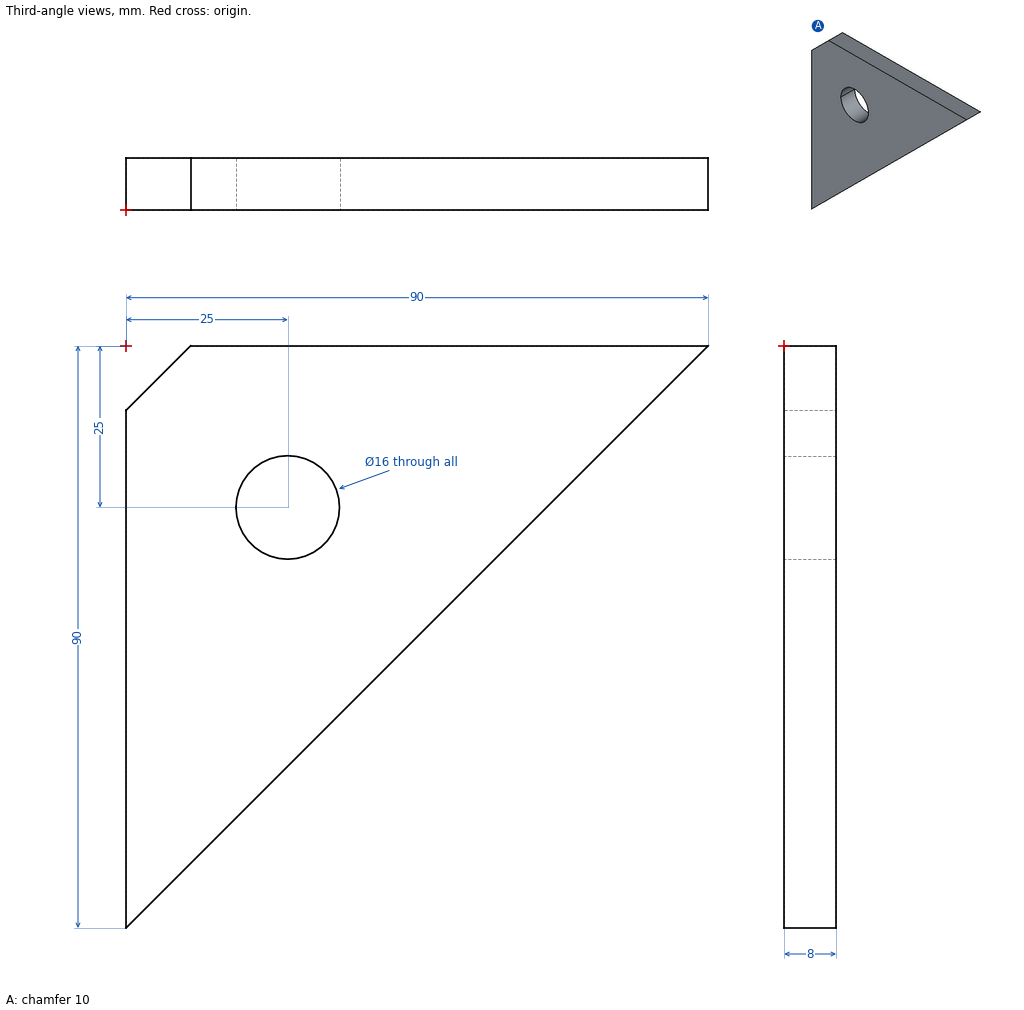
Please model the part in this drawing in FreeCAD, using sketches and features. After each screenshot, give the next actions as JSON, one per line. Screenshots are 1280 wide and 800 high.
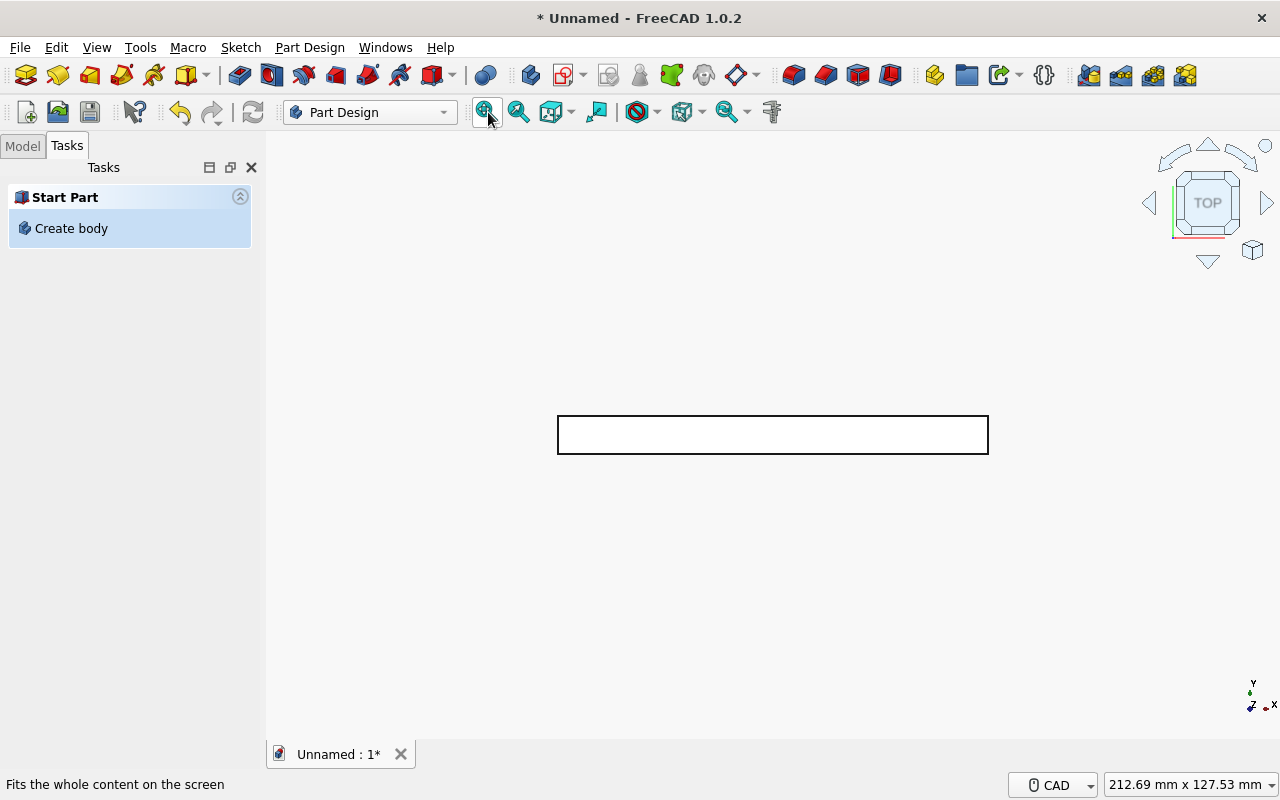
{"action": "left_click", "coordinate": [488, 112]}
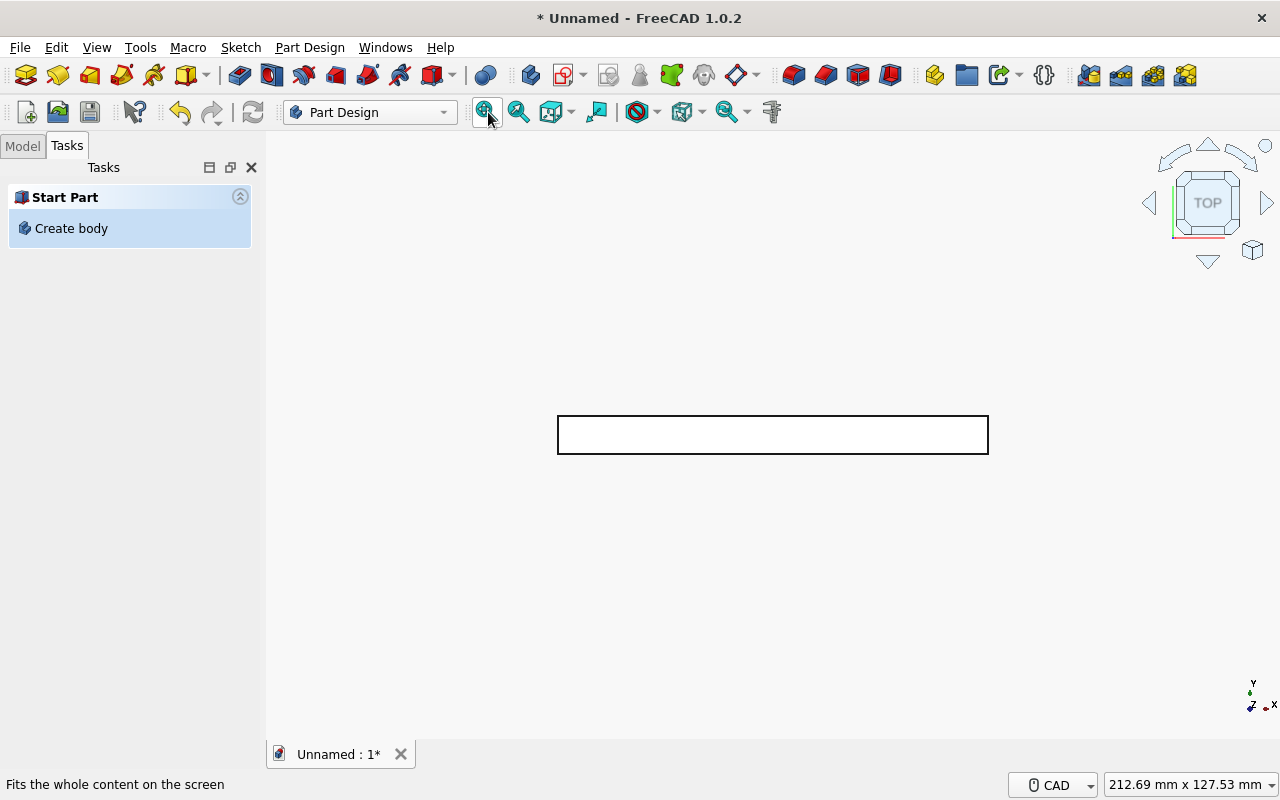
{"action": "left_click", "coordinate": [558, 423]}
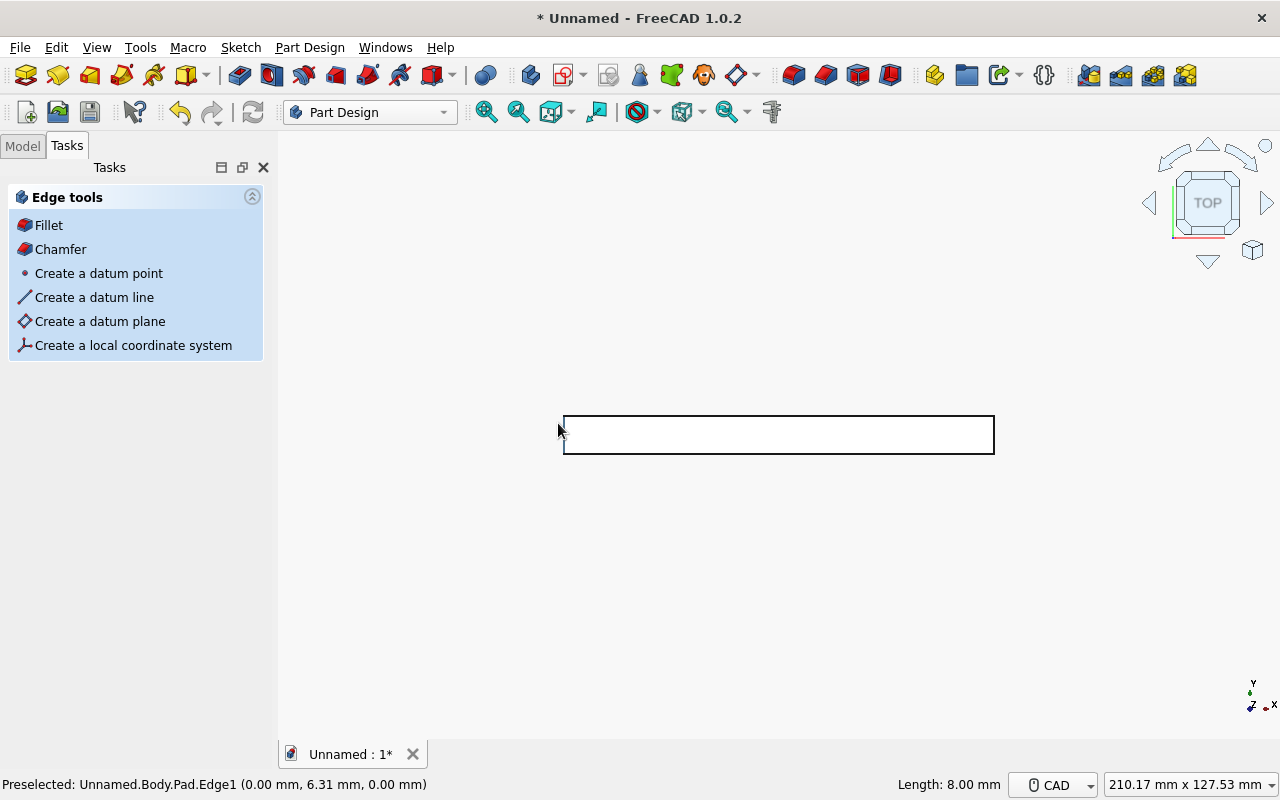
{"action": "left_click", "coordinate": [826, 76]}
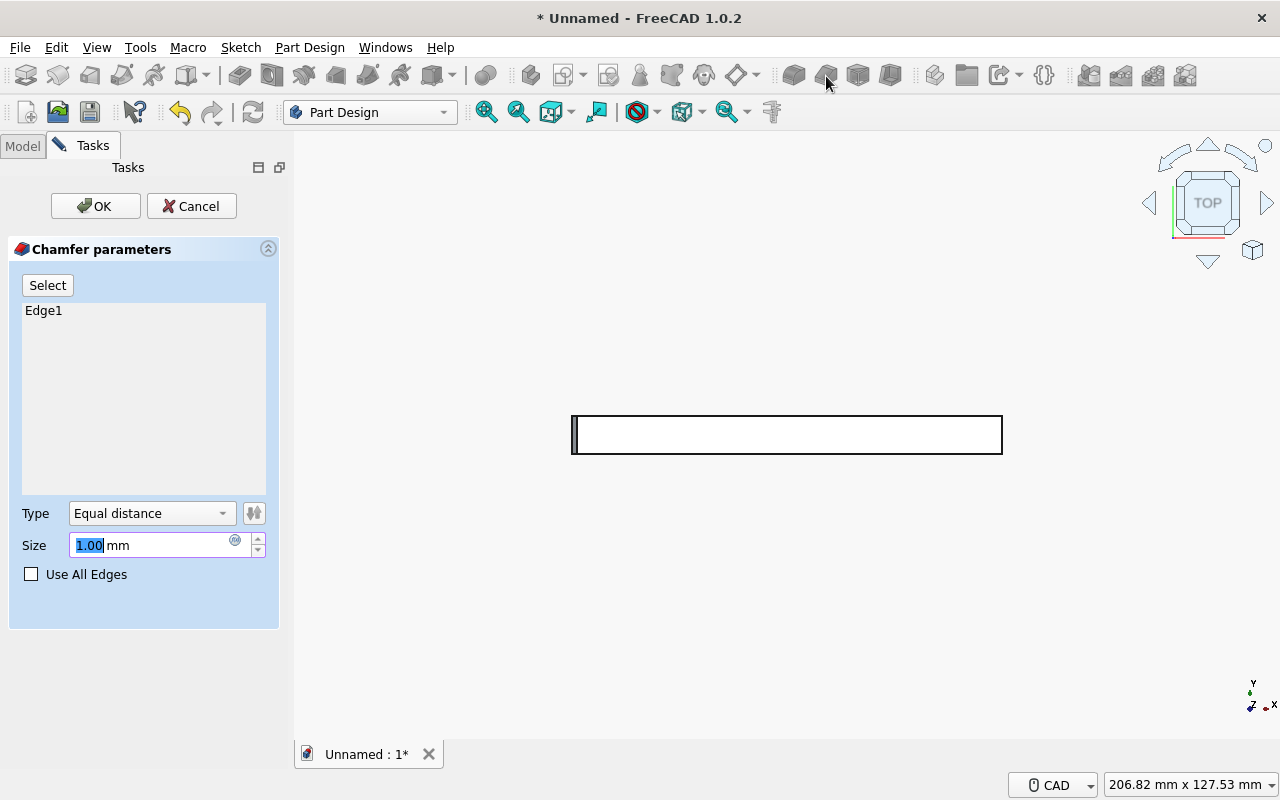
{"action": "type", "text": "10"}
{"action": "key", "text": "Tab"}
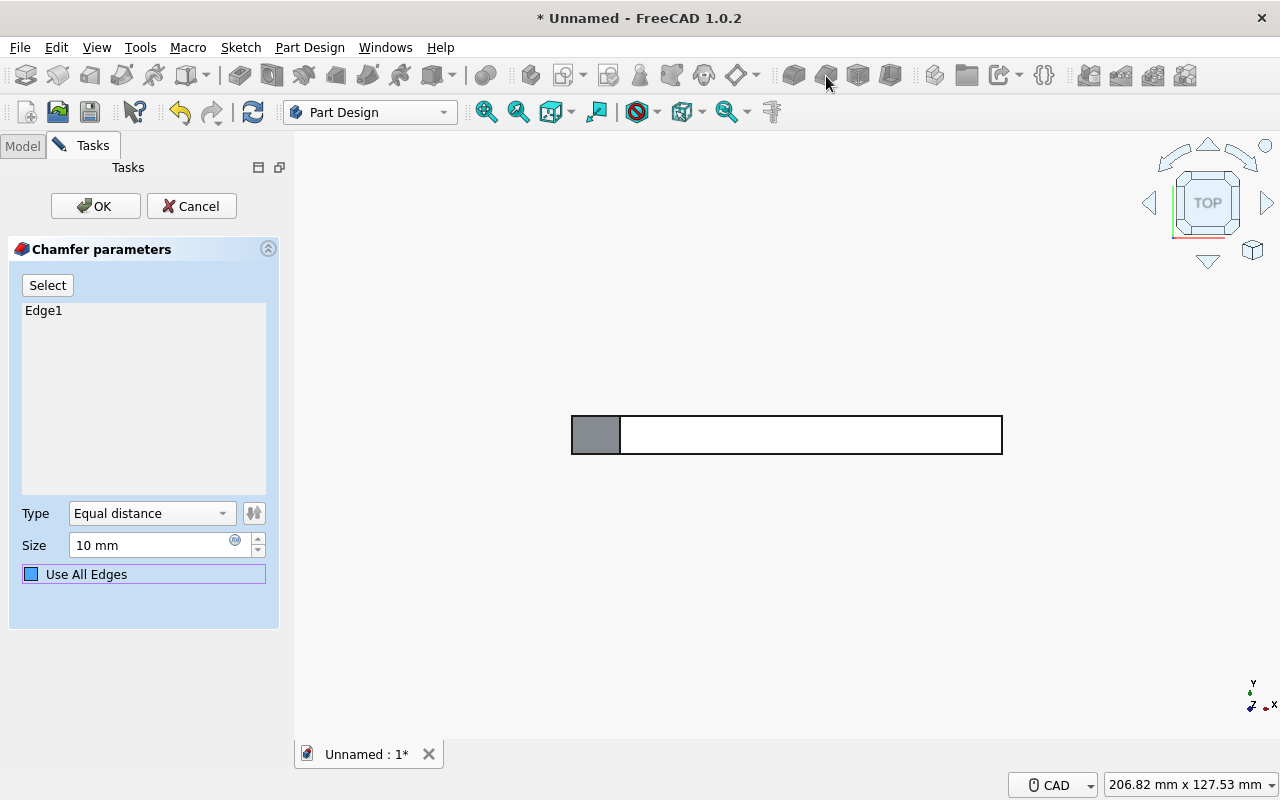
{"action": "left_click", "coordinate": [96, 206]}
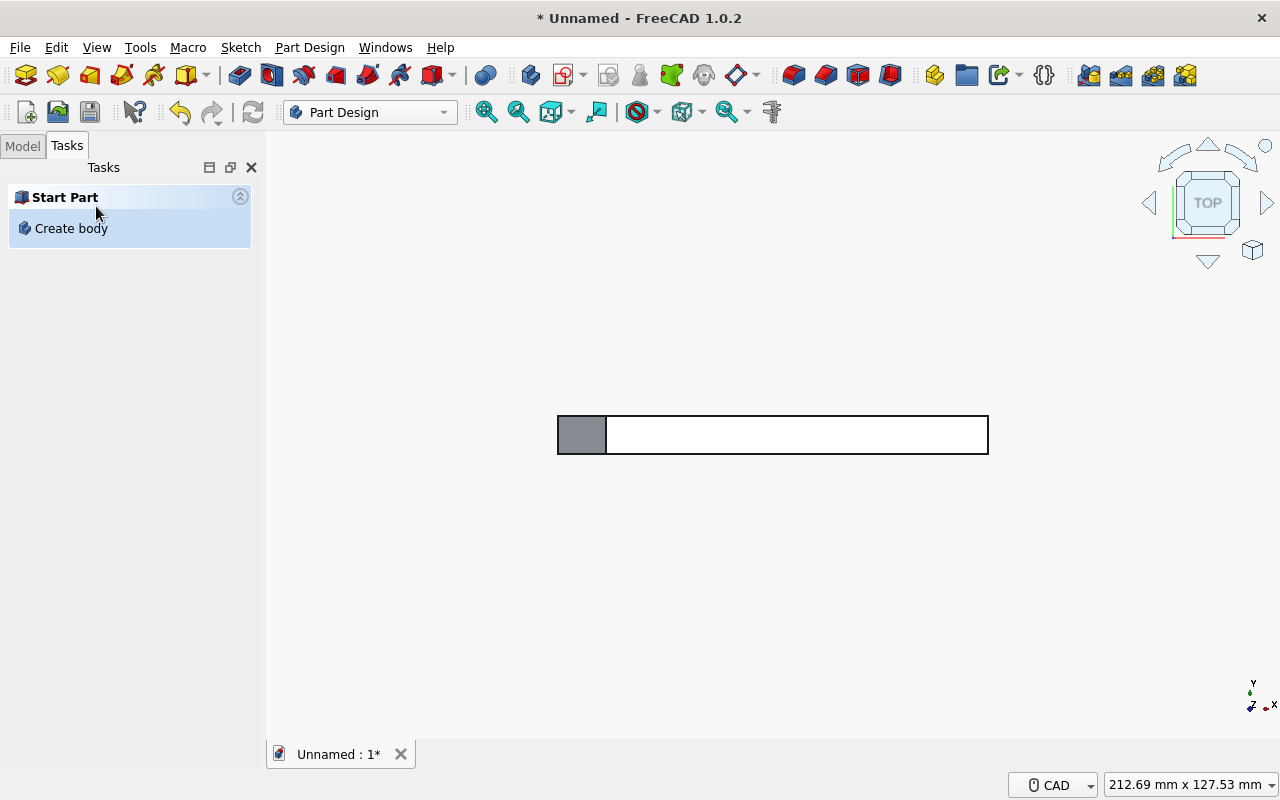
{"action": "key", "text": "v f"}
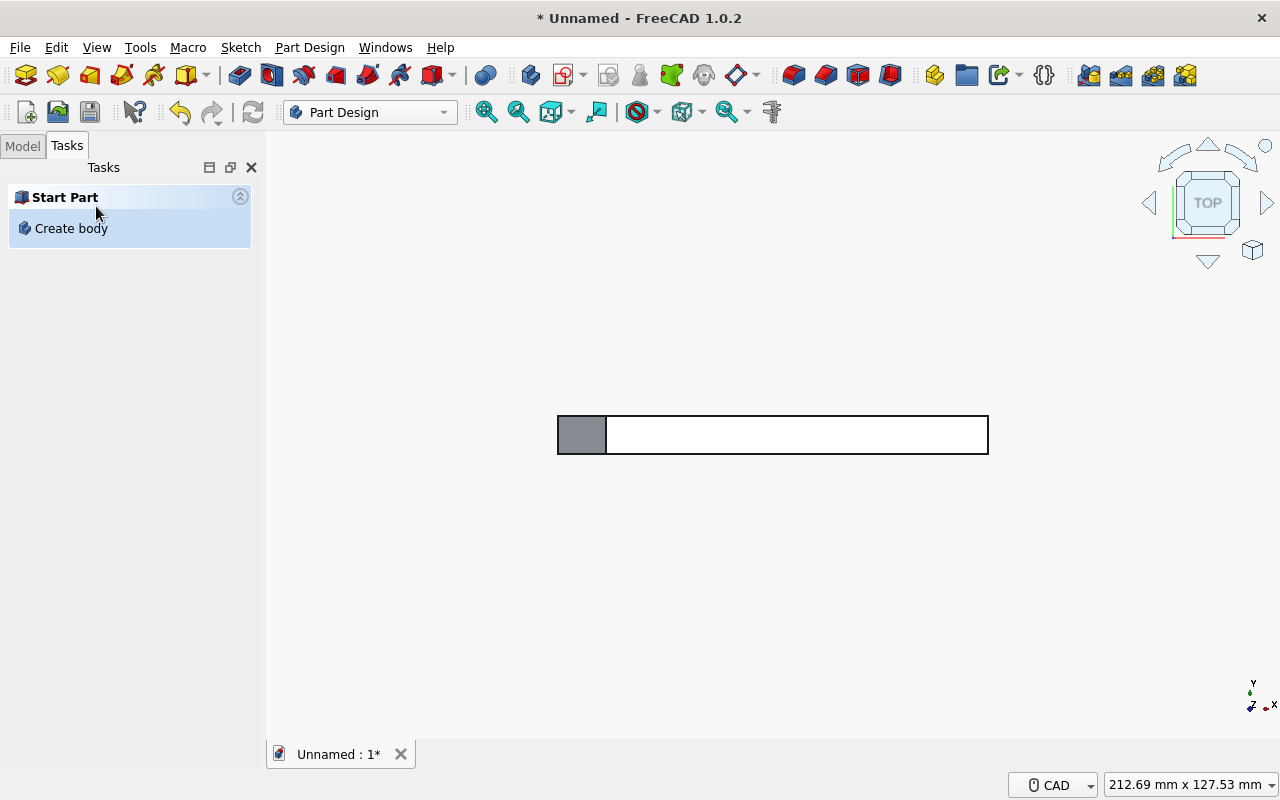
{"action": "key", "text": "4"}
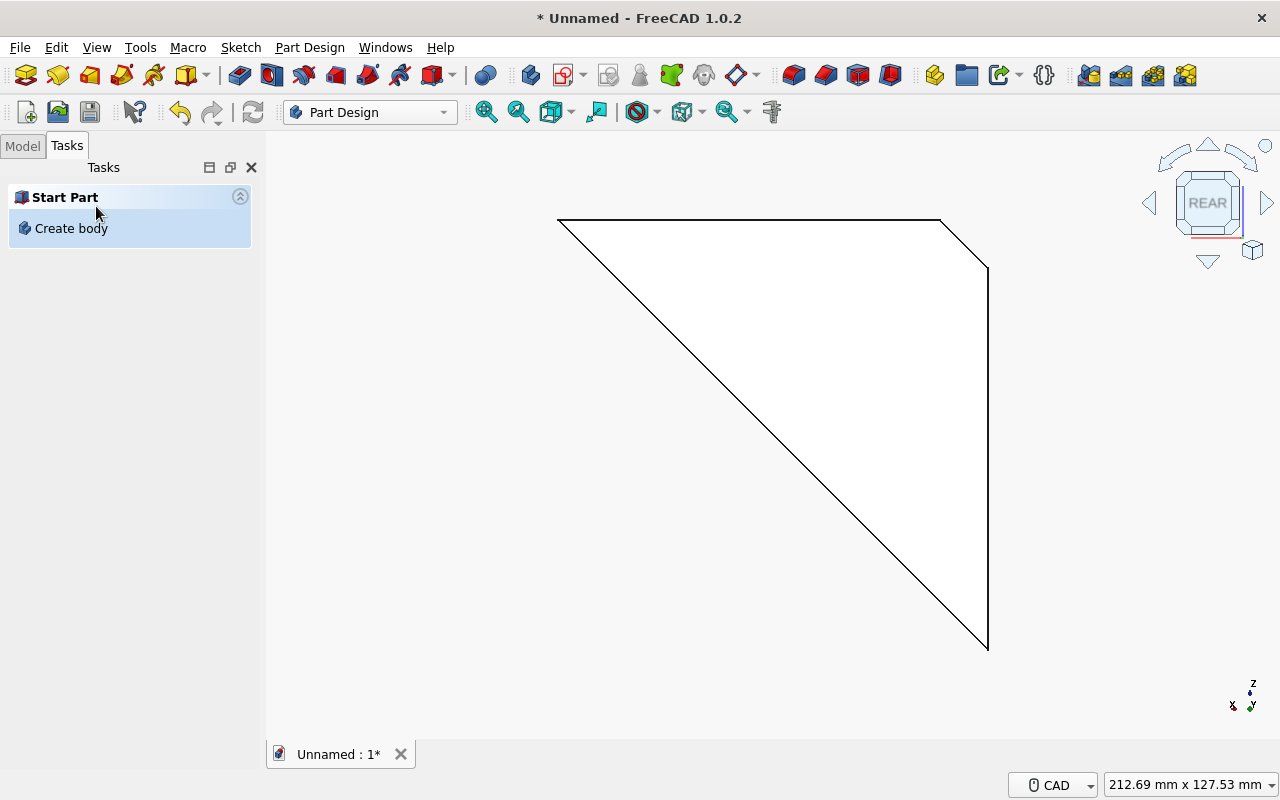
{"action": "left_click", "coordinate": [834, 311]}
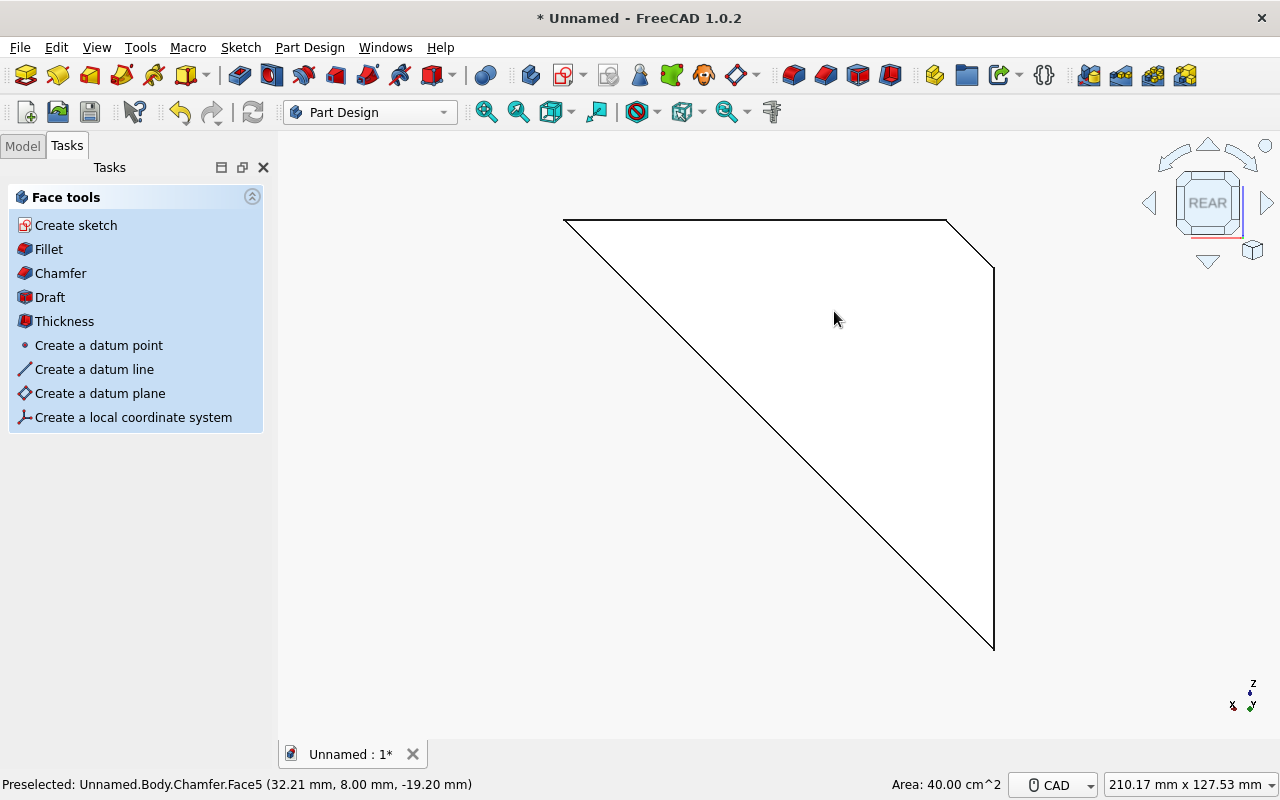
{"action": "left_click", "coordinate": [564, 76]}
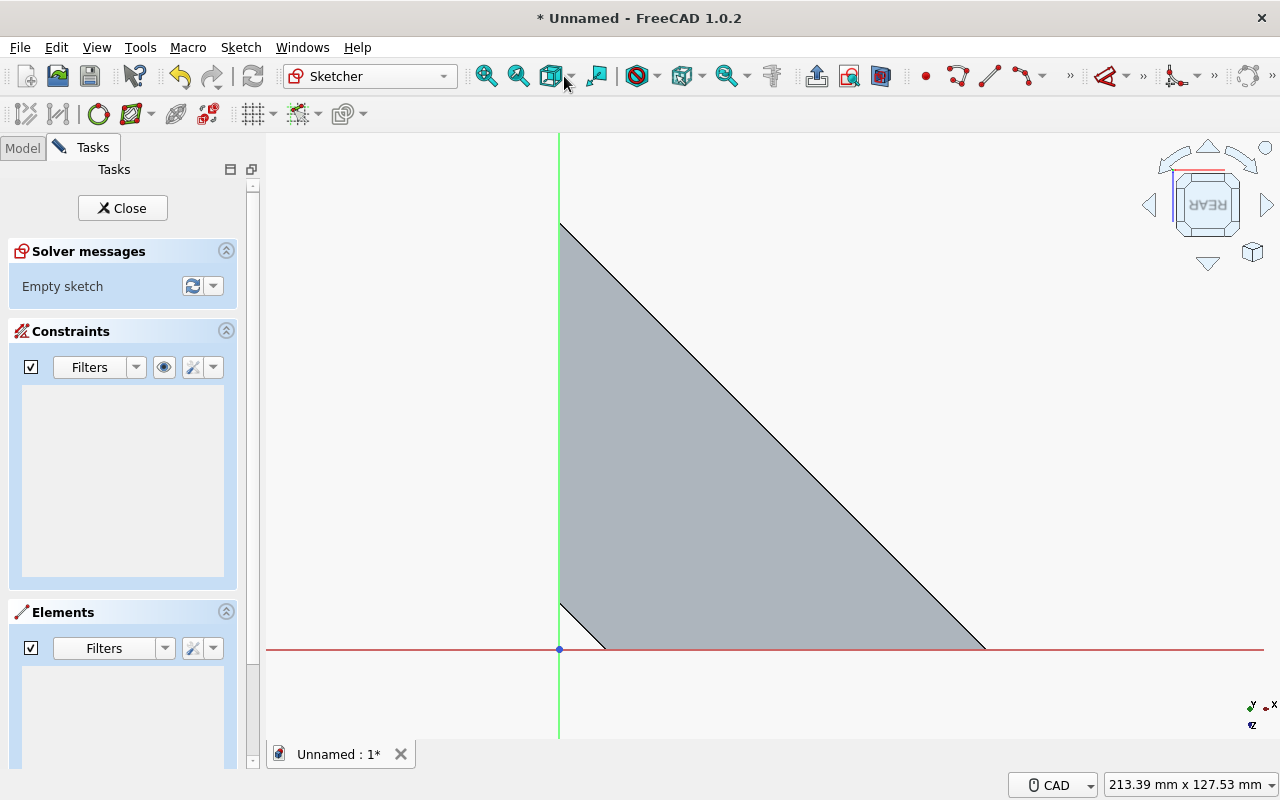
{"action": "scroll", "coordinate": [599, 650], "scroll_direction": "up", "scroll_amount": 5}